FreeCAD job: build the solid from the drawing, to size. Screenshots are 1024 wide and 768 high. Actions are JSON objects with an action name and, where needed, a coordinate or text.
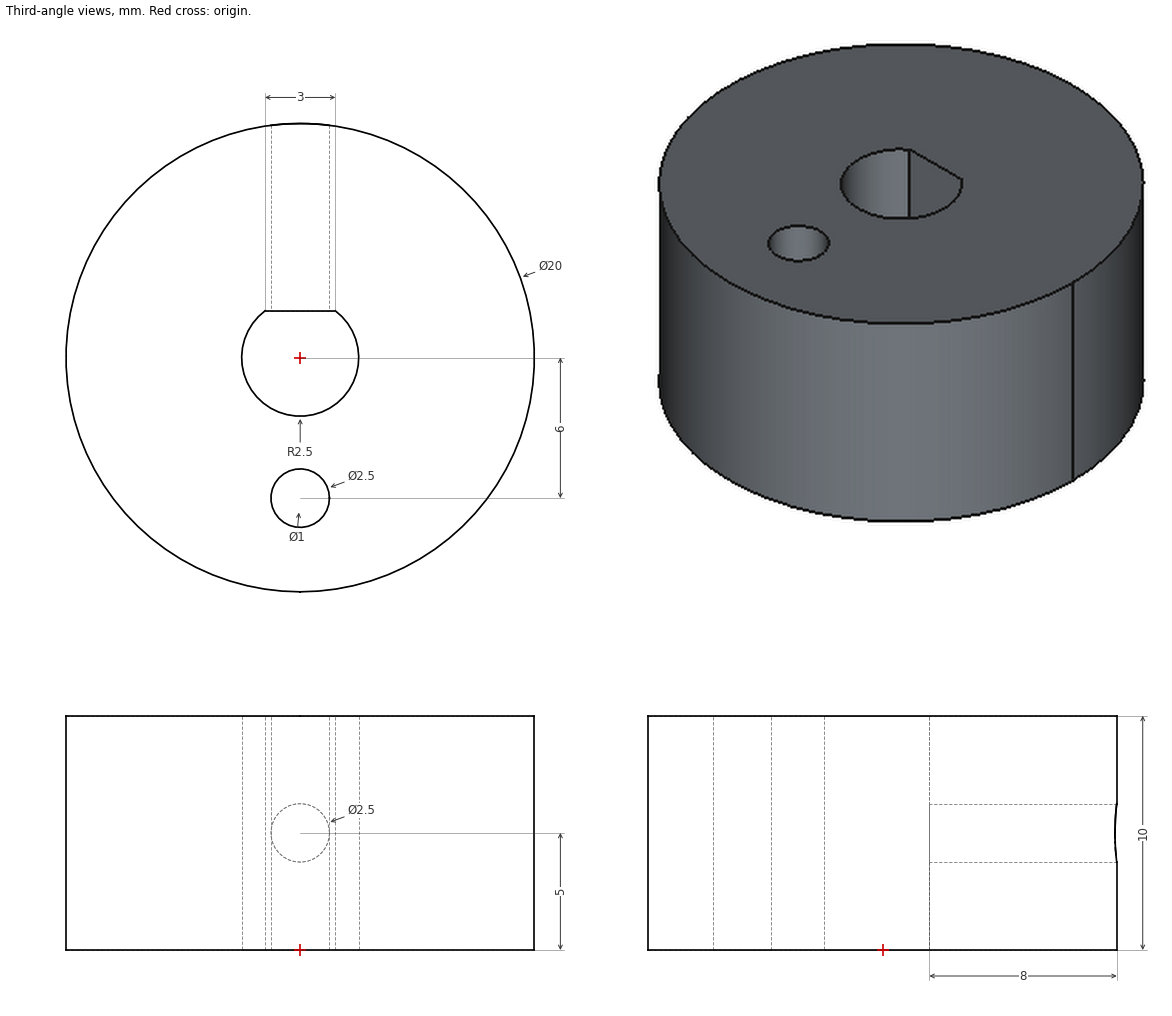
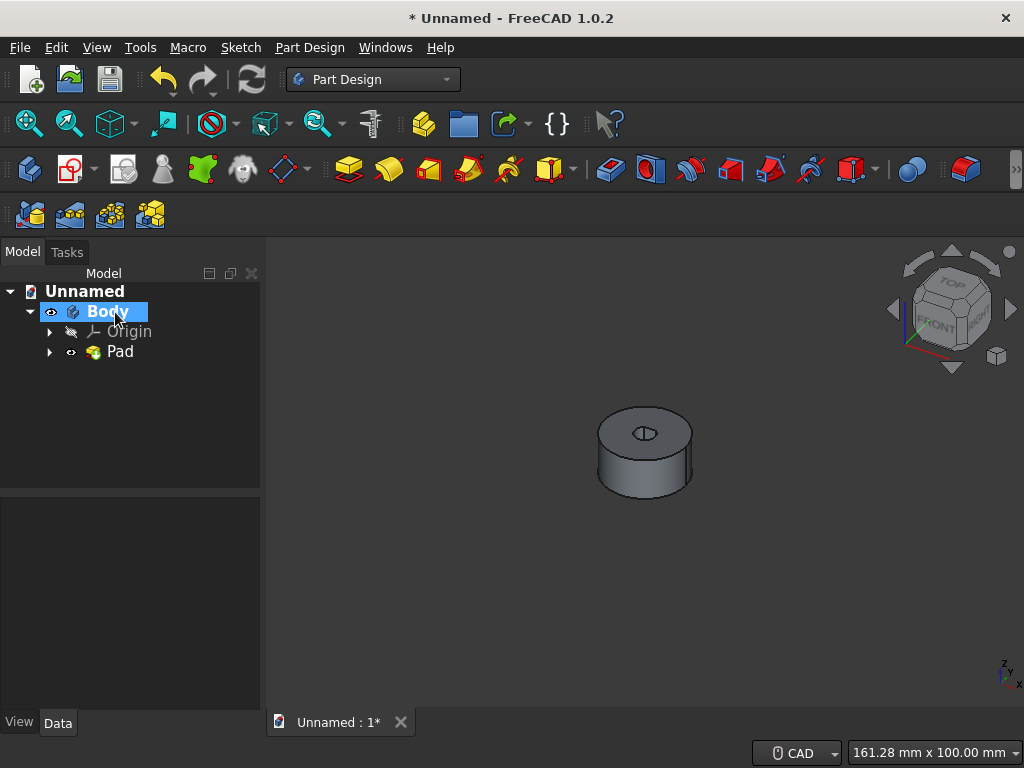
{"action": "left_click", "coordinate": [30, 124]}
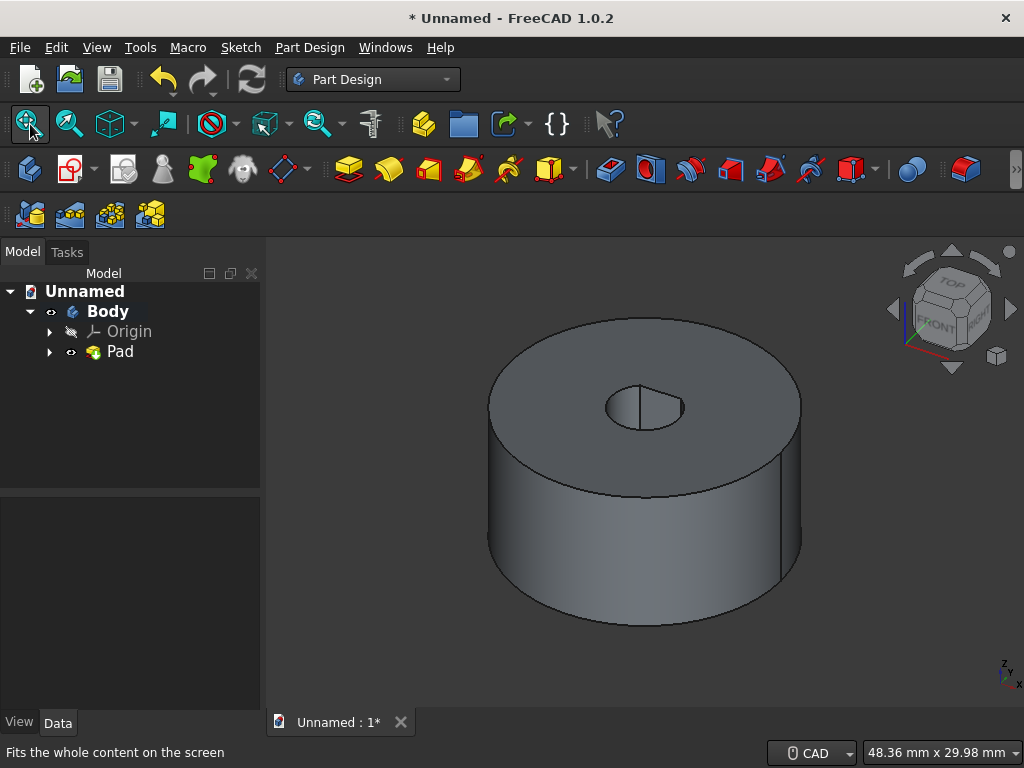
{"action": "left_click", "coordinate": [690, 362]}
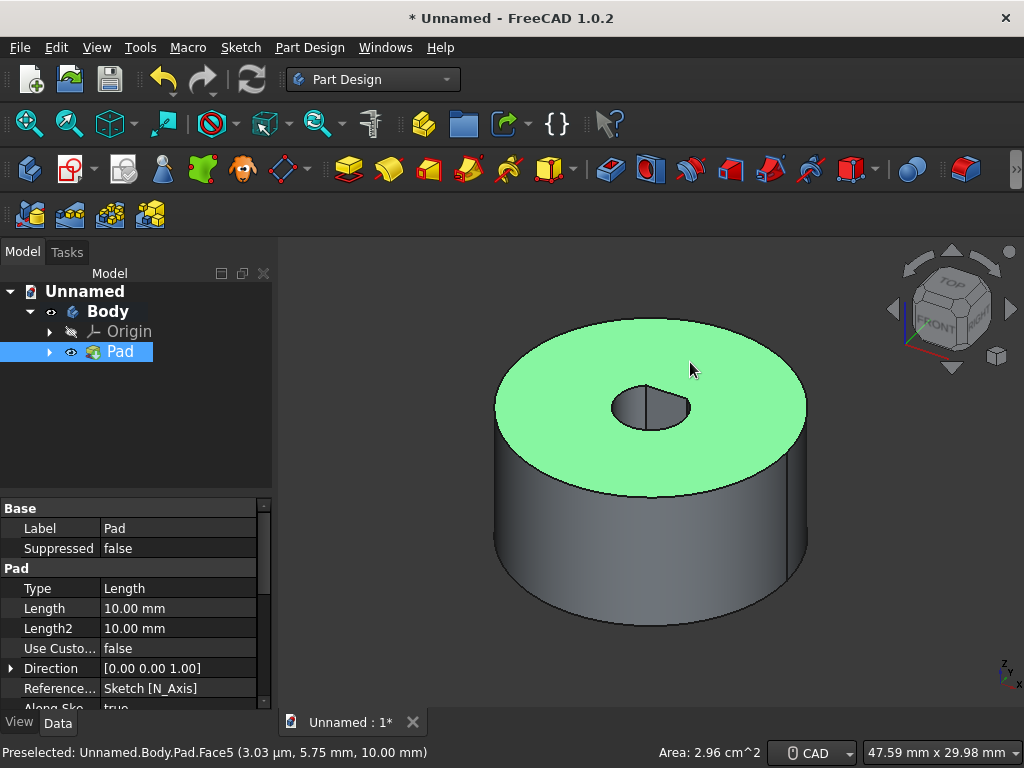
{"action": "left_click", "coordinate": [70, 170]}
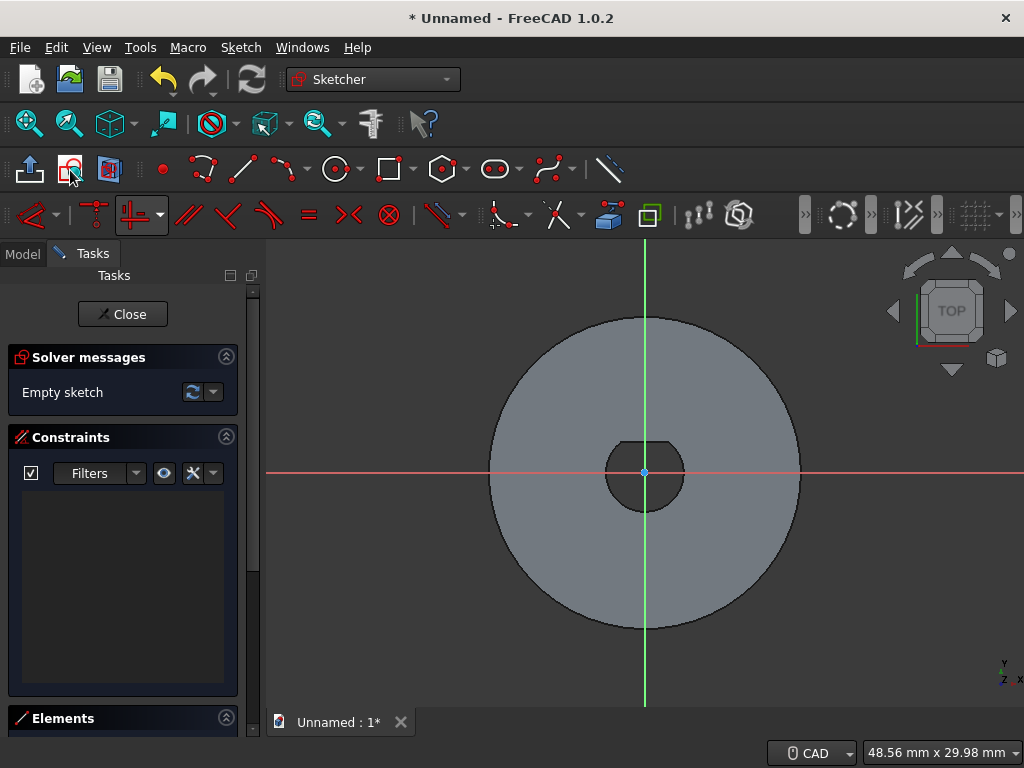
{"action": "scroll", "coordinate": [648, 572], "scroll_direction": "up", "scroll_amount": 15}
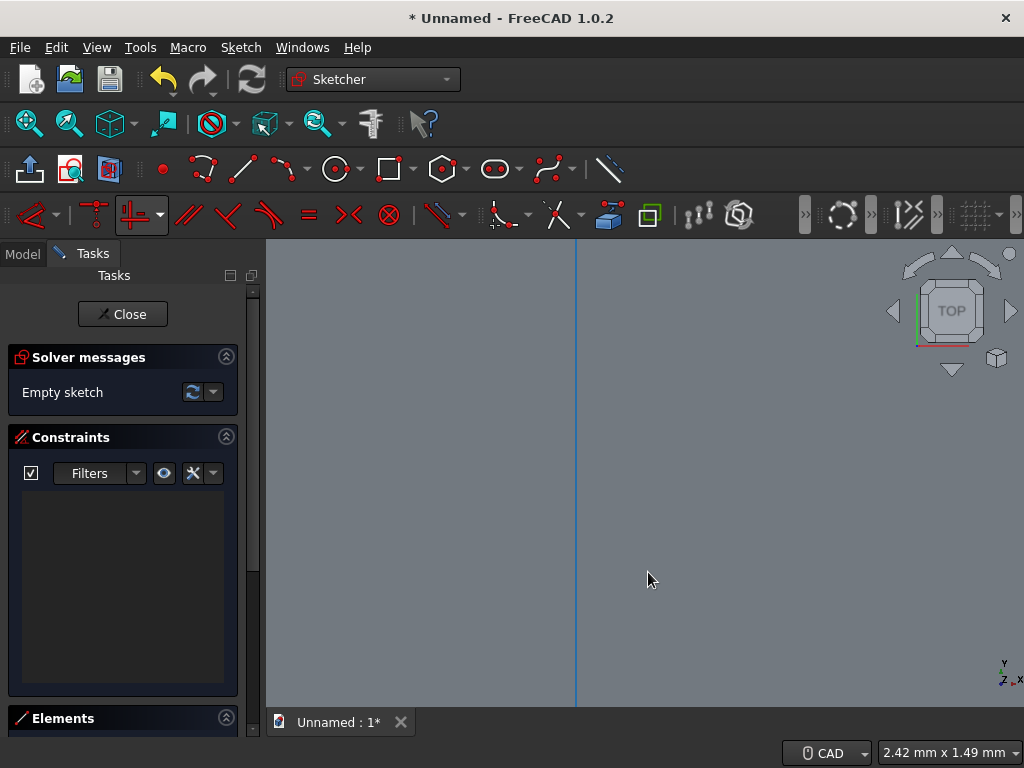
{"action": "key", "text": "g c"}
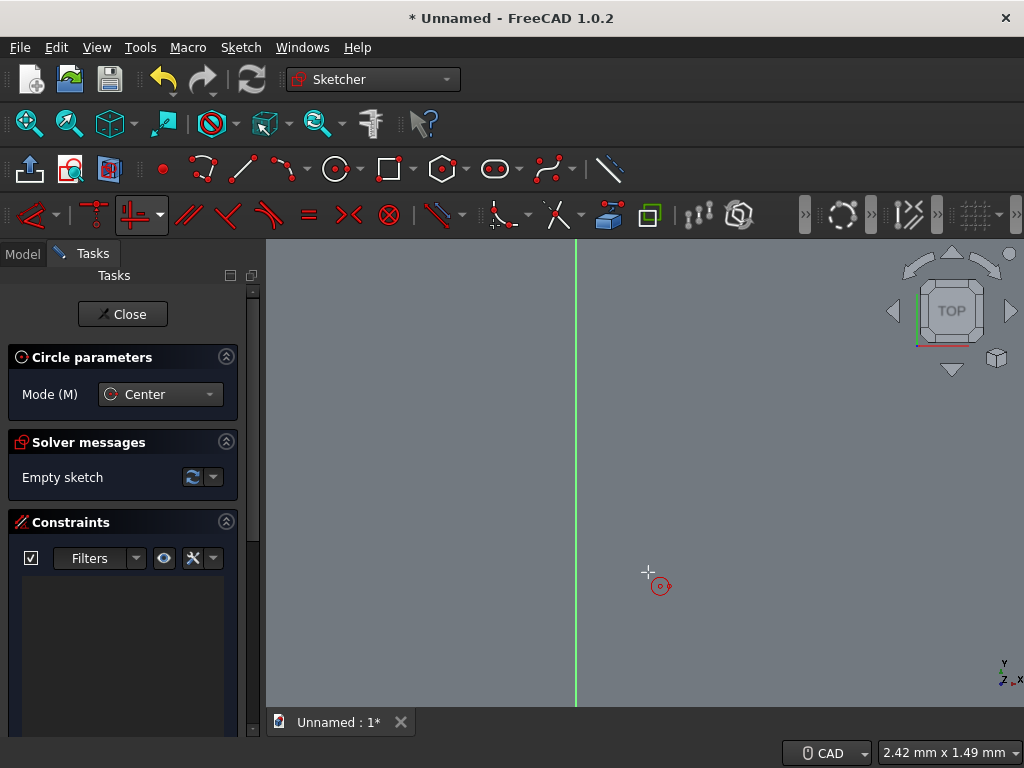
{"action": "left_click", "coordinate": [576, 451]}
{"action": "mouse_move", "coordinate": [686, 340]}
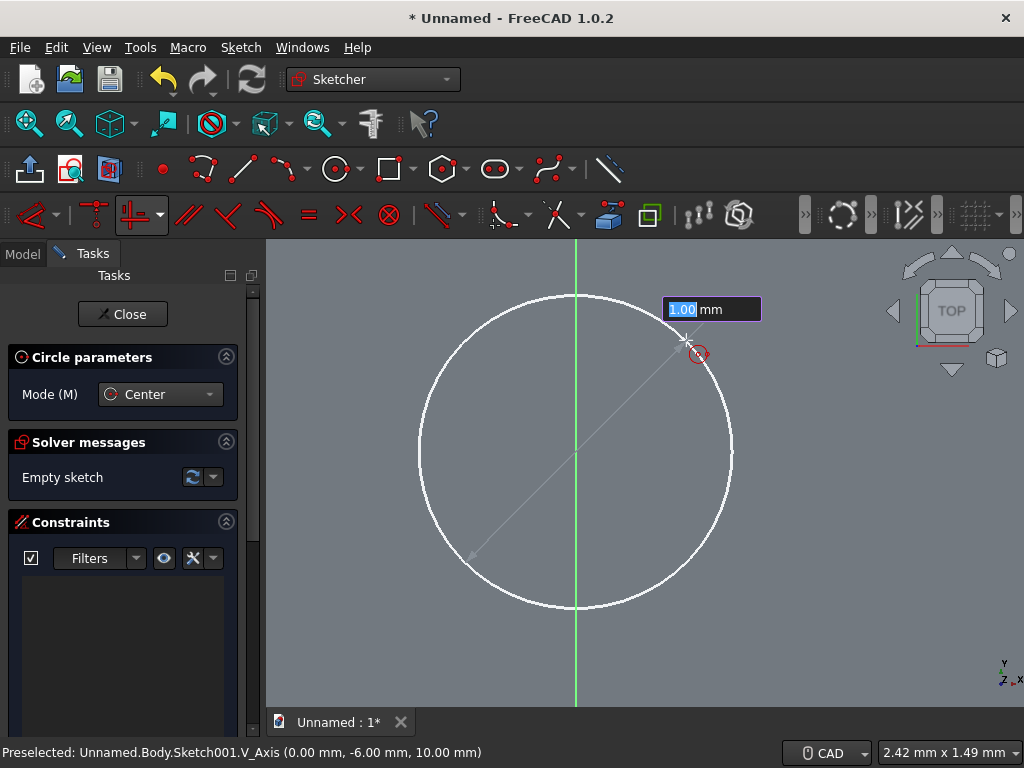
{"action": "type", "text": "1"}
{"action": "key", "text": "Return"}
{"action": "key", "text": "Escape"}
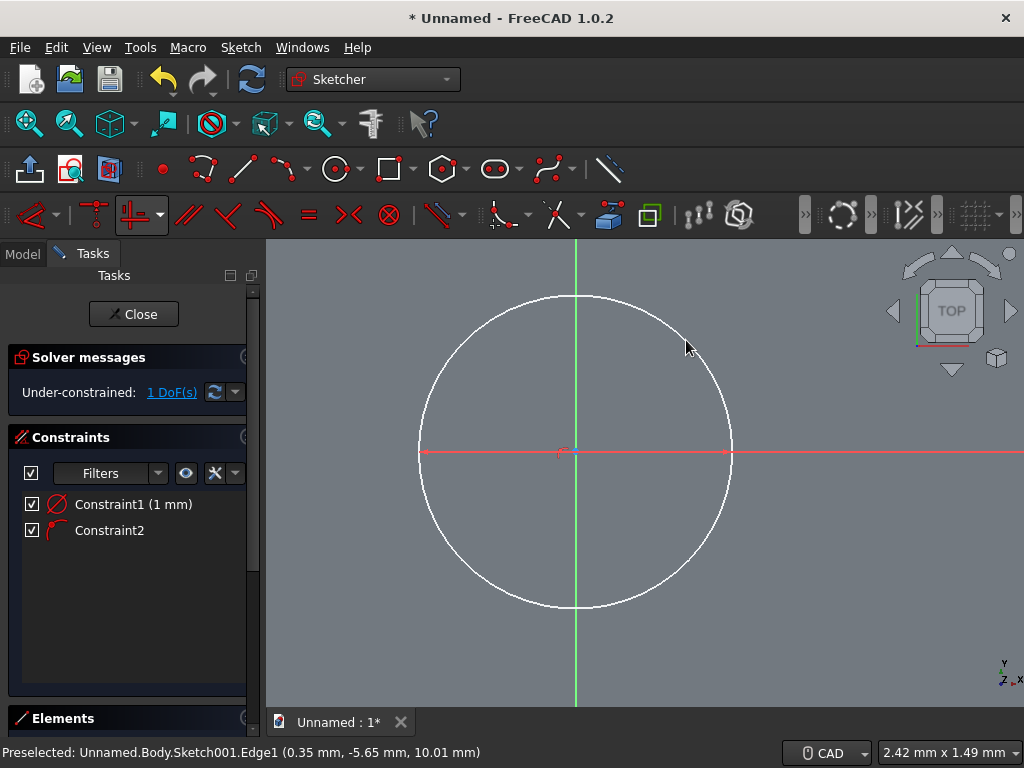
{"action": "key", "text": "d"}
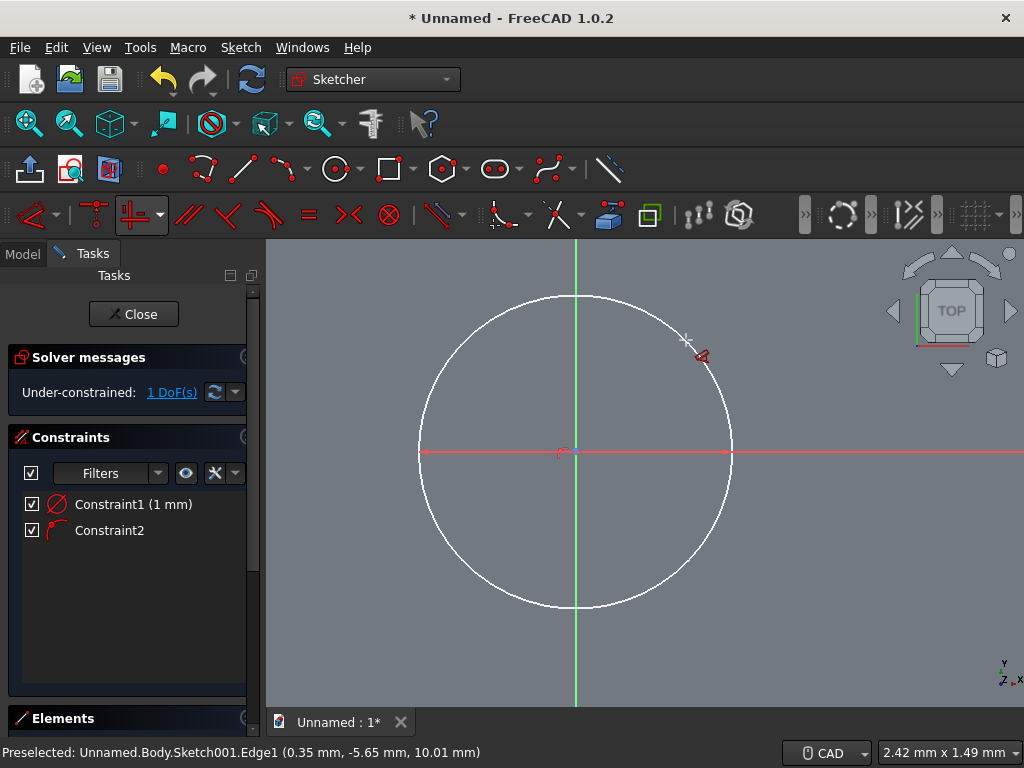
{"action": "left_click", "coordinate": [576, 452]}
{"action": "left_click", "coordinate": [610, 360]}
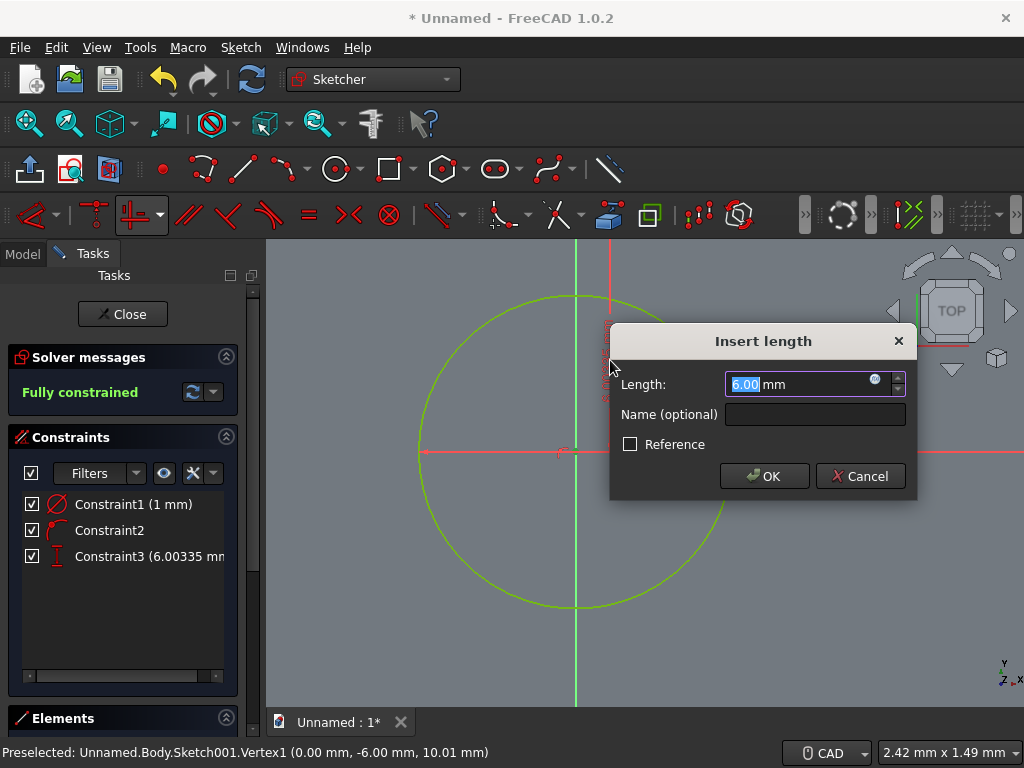
{"action": "type", "text": "6"}
{"action": "key", "text": "Return"}
{"action": "key", "text": "Escape"}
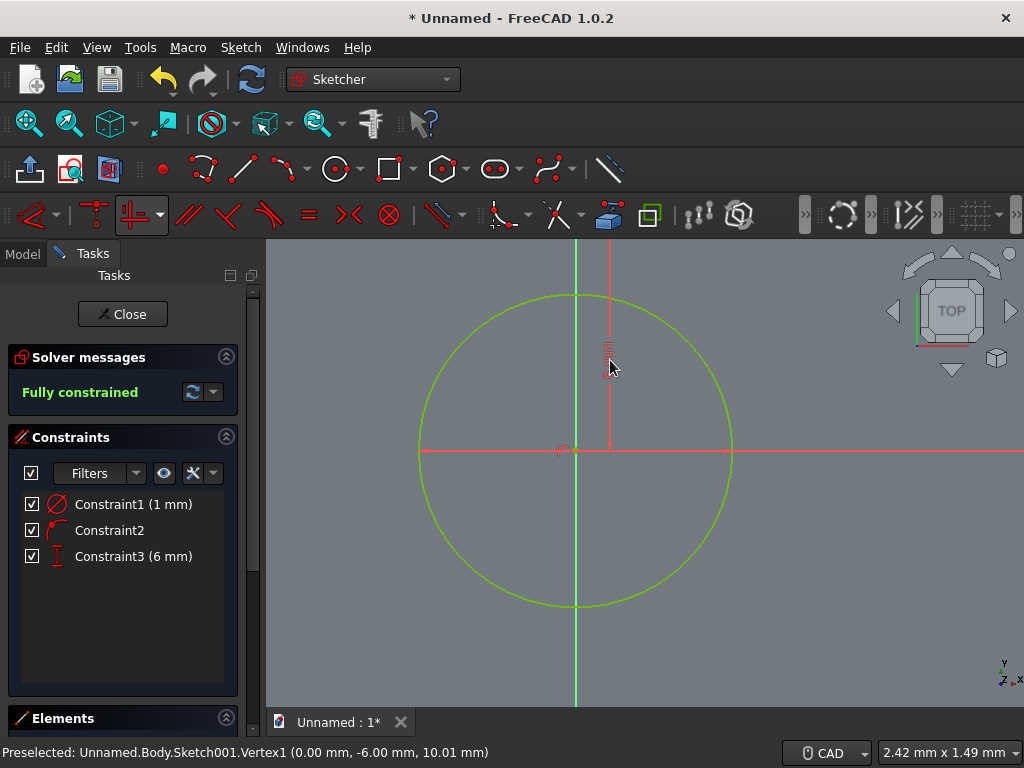
{"action": "left_click", "coordinate": [123, 314]}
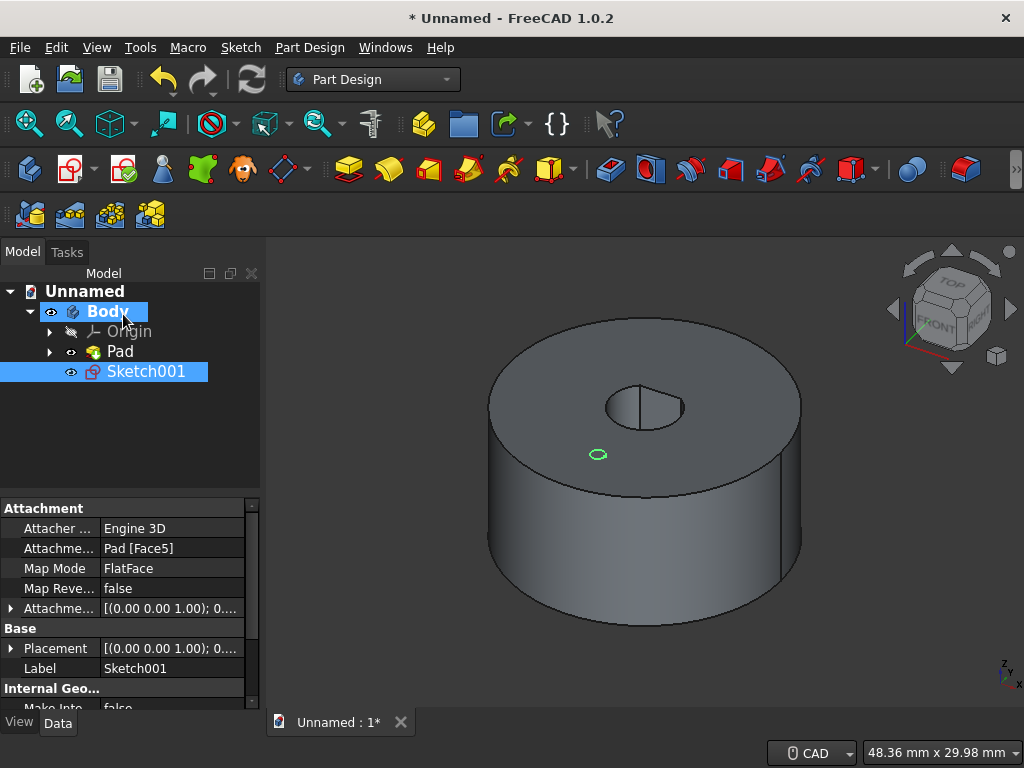
{"action": "left_click", "coordinate": [612, 170]}